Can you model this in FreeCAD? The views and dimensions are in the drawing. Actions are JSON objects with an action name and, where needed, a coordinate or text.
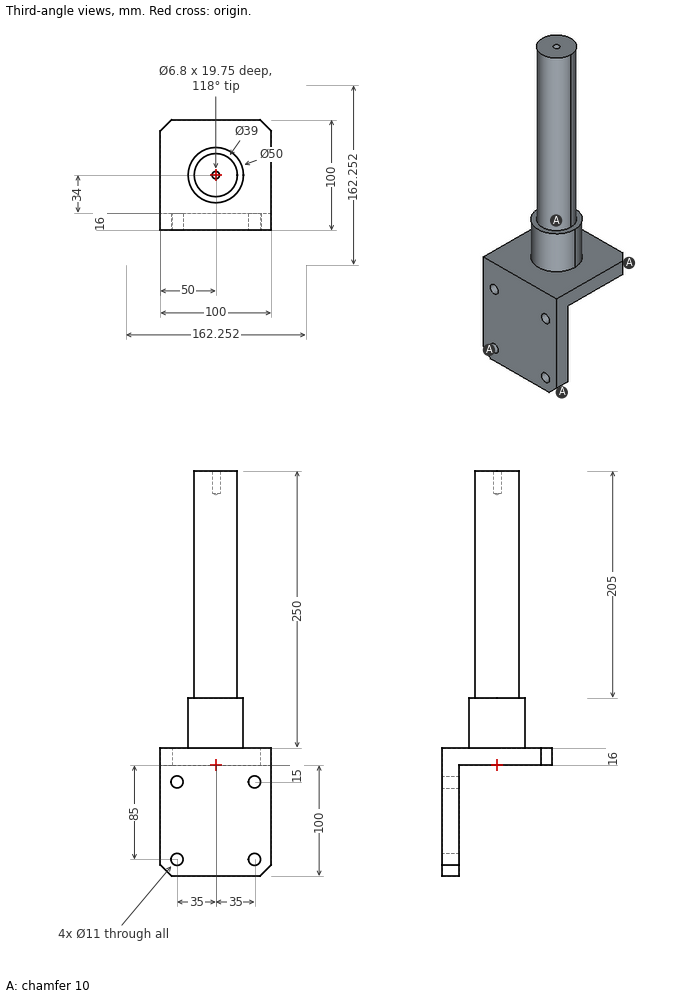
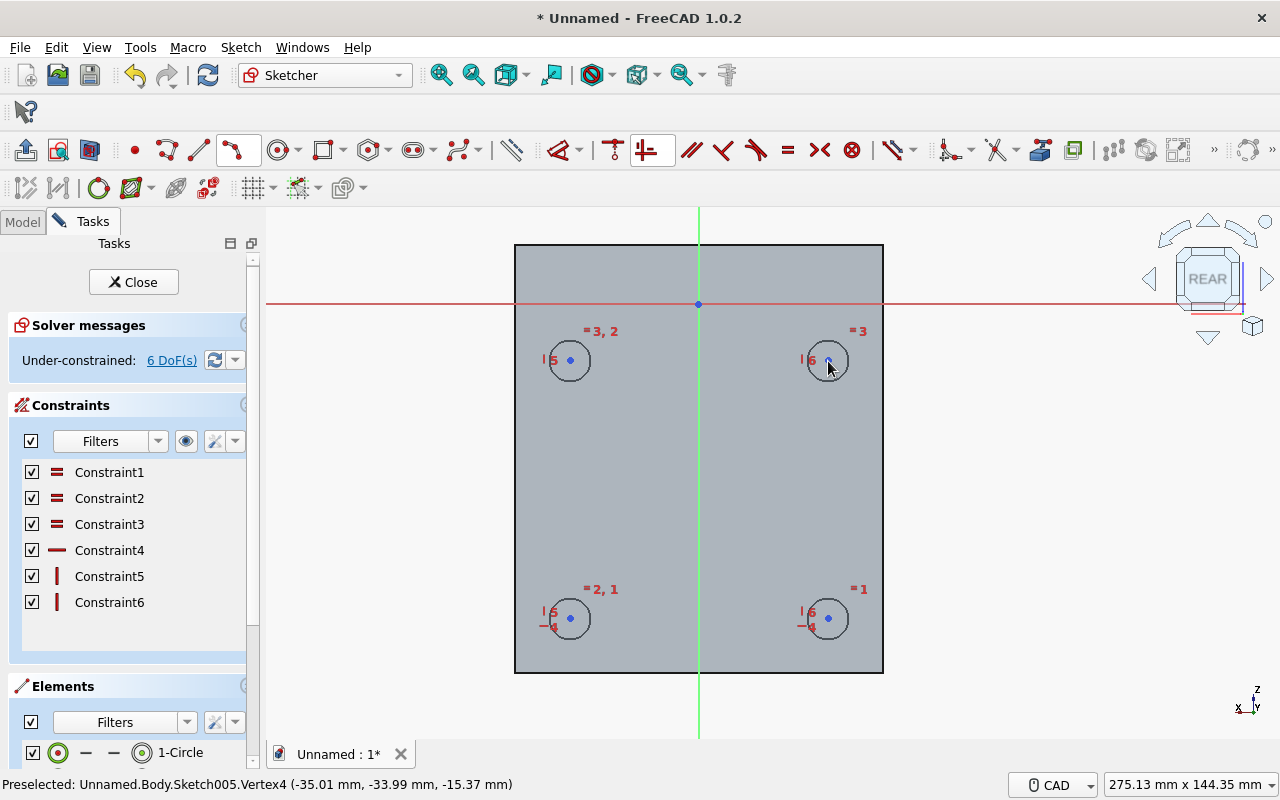
{"action": "left_click", "coordinate": [570, 361]}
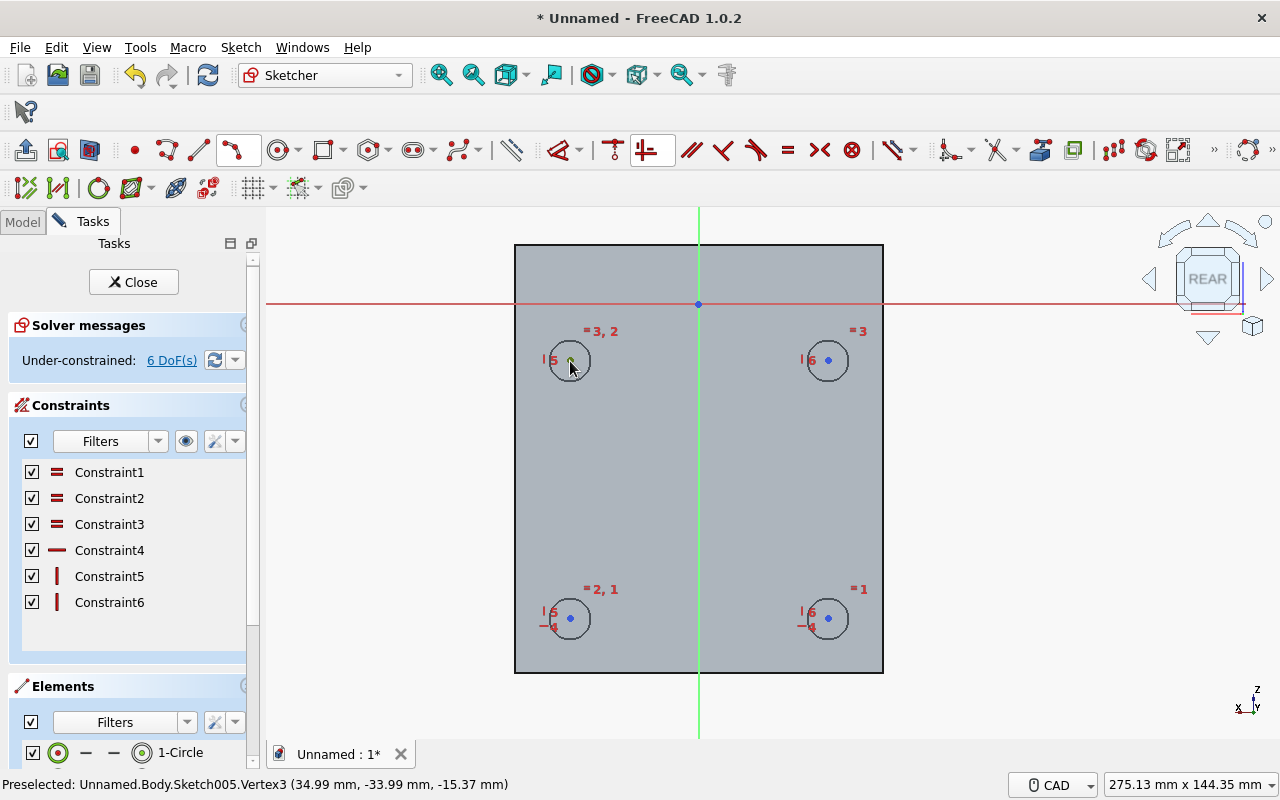
{"action": "left_click", "coordinate": [828, 361]}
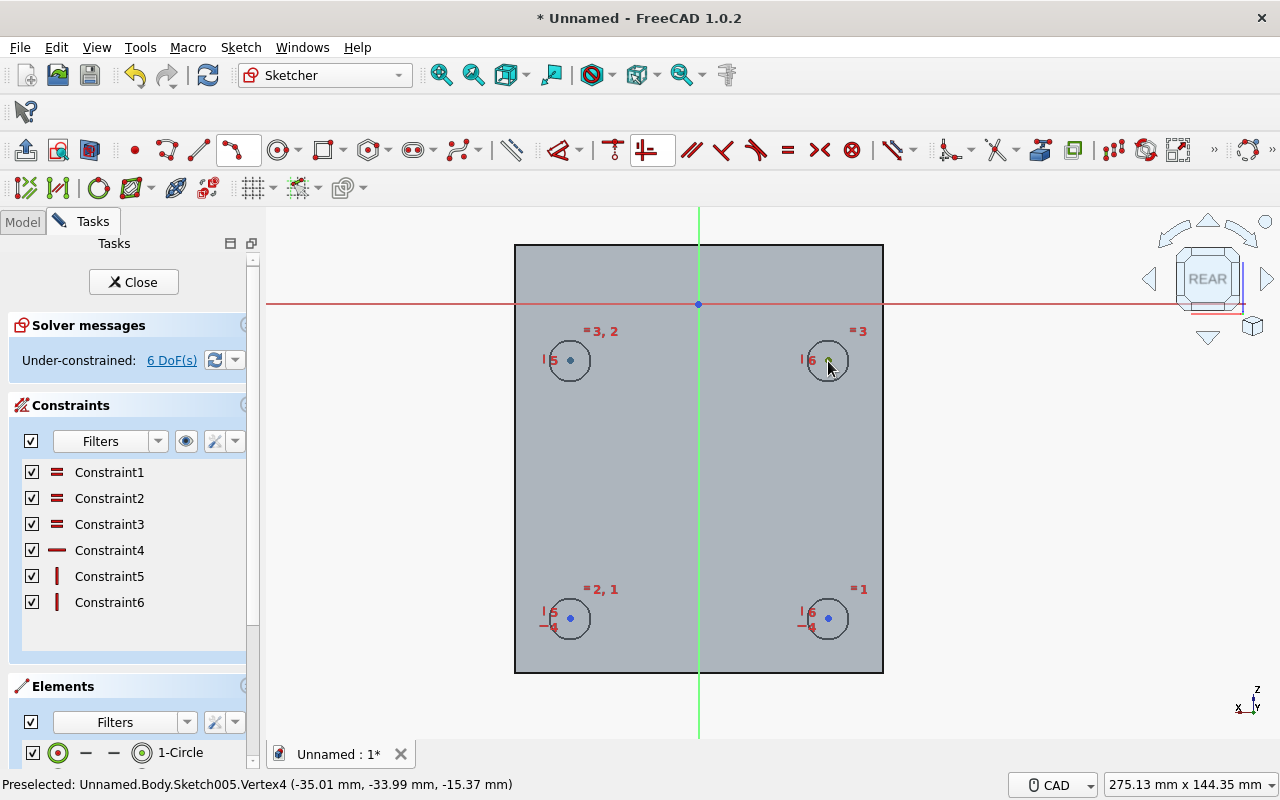
{"action": "key", "text": "h"}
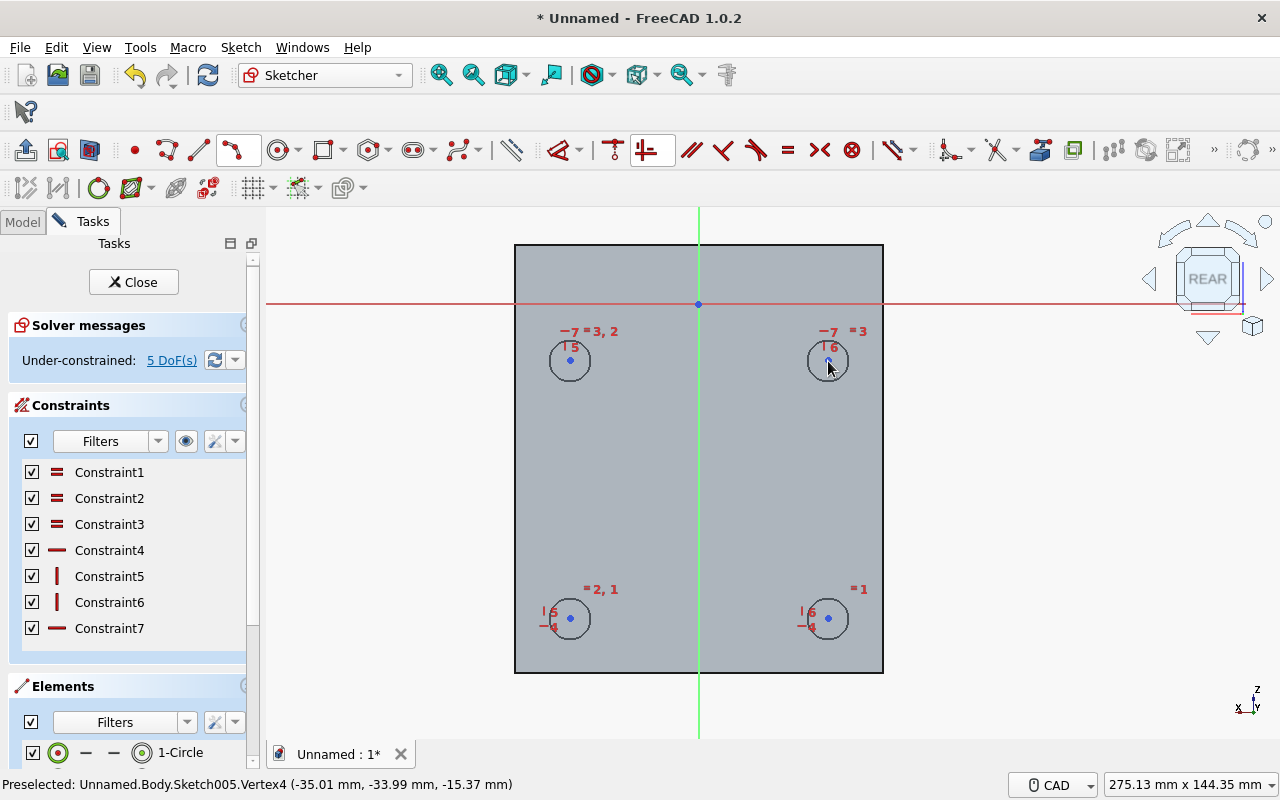
{"action": "left_click", "coordinate": [558, 150]}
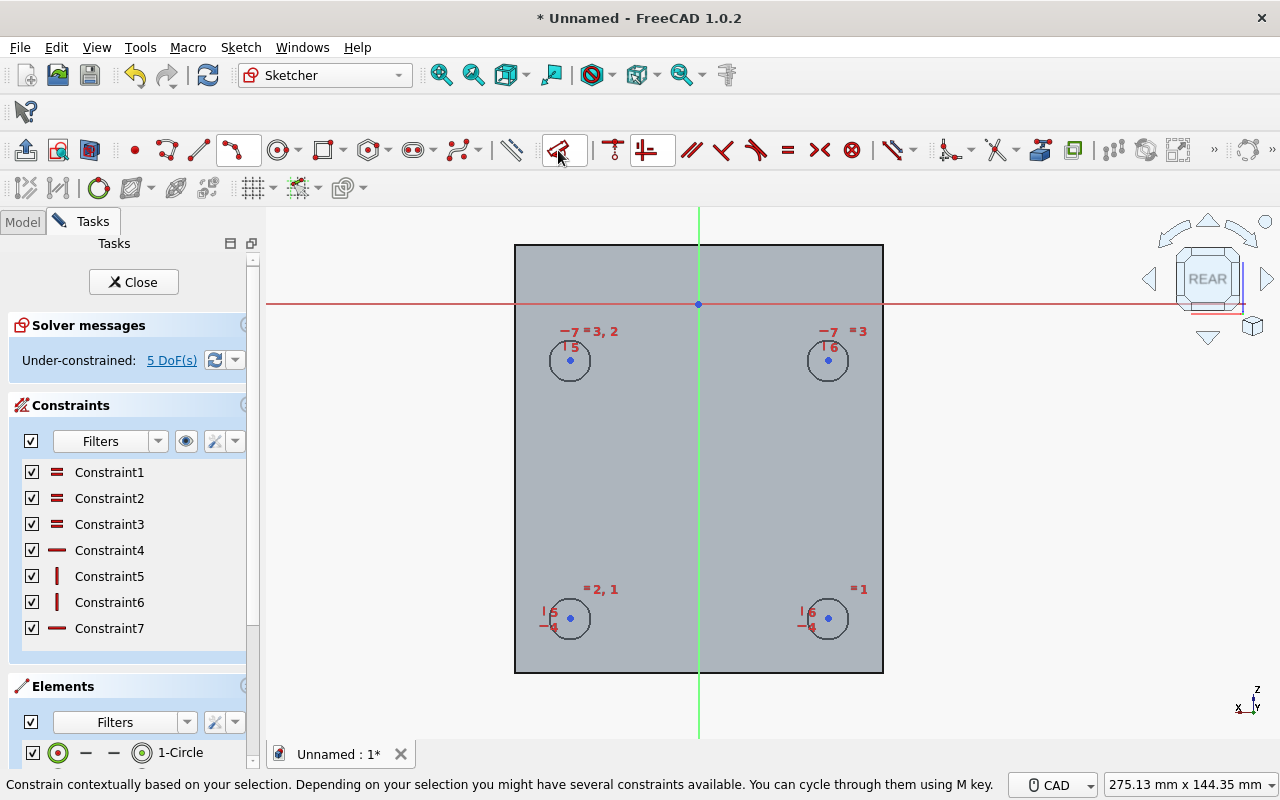
{"action": "left_click", "coordinate": [842, 604]}
{"action": "left_click", "coordinate": [864, 581]}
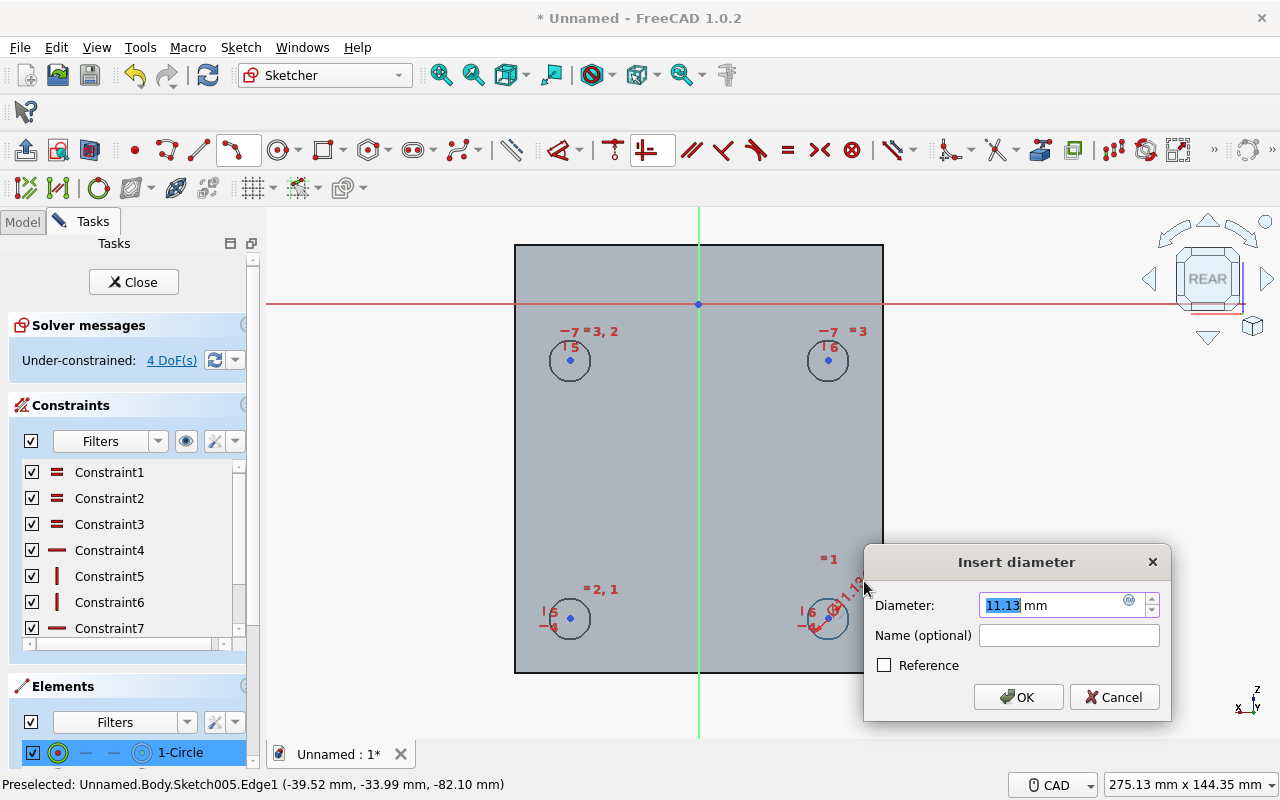
{"action": "type", "text": "11"}
{"action": "key", "text": "Return"}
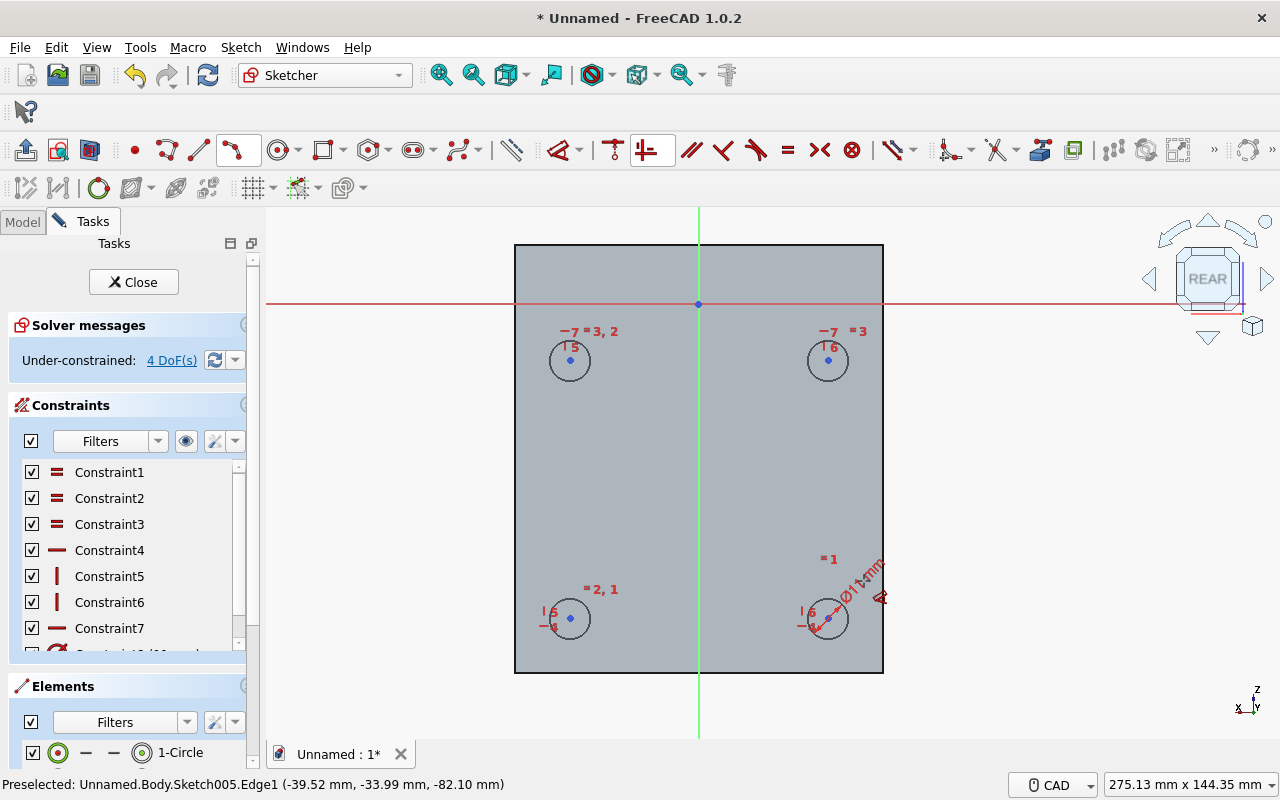
{"action": "left_click", "coordinate": [828, 619]}
{"action": "left_click", "coordinate": [763, 270]}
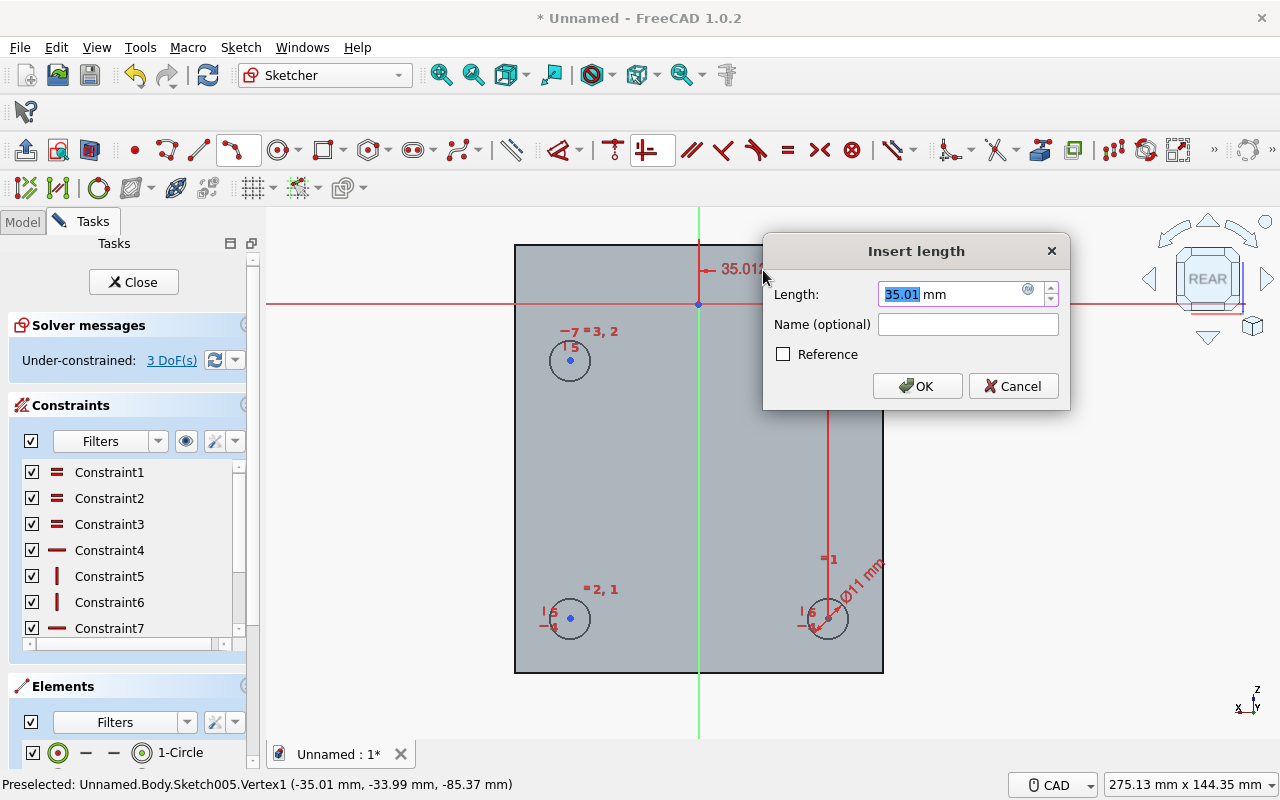
{"action": "type", "text": "35"}
{"action": "key", "text": "Return"}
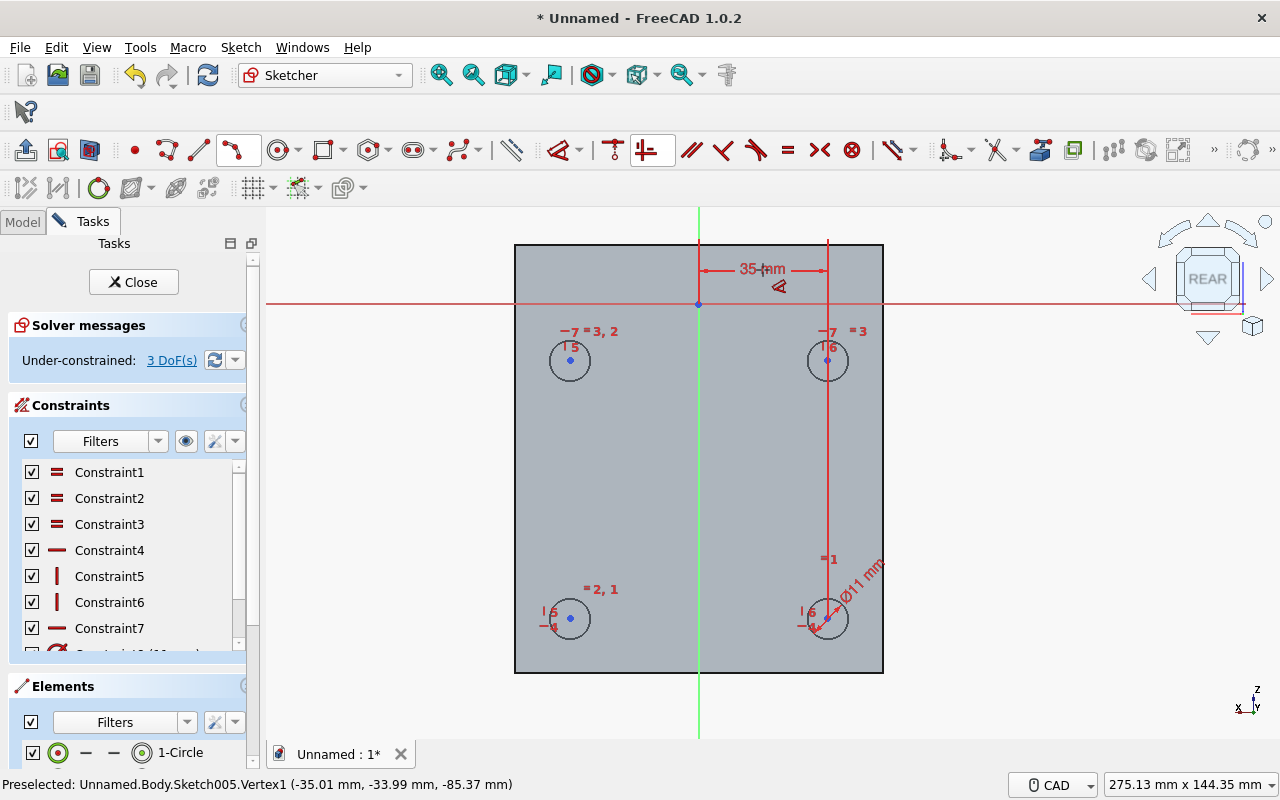
{"action": "left_click", "coordinate": [828, 619]}
{"action": "left_click", "coordinate": [862, 462]}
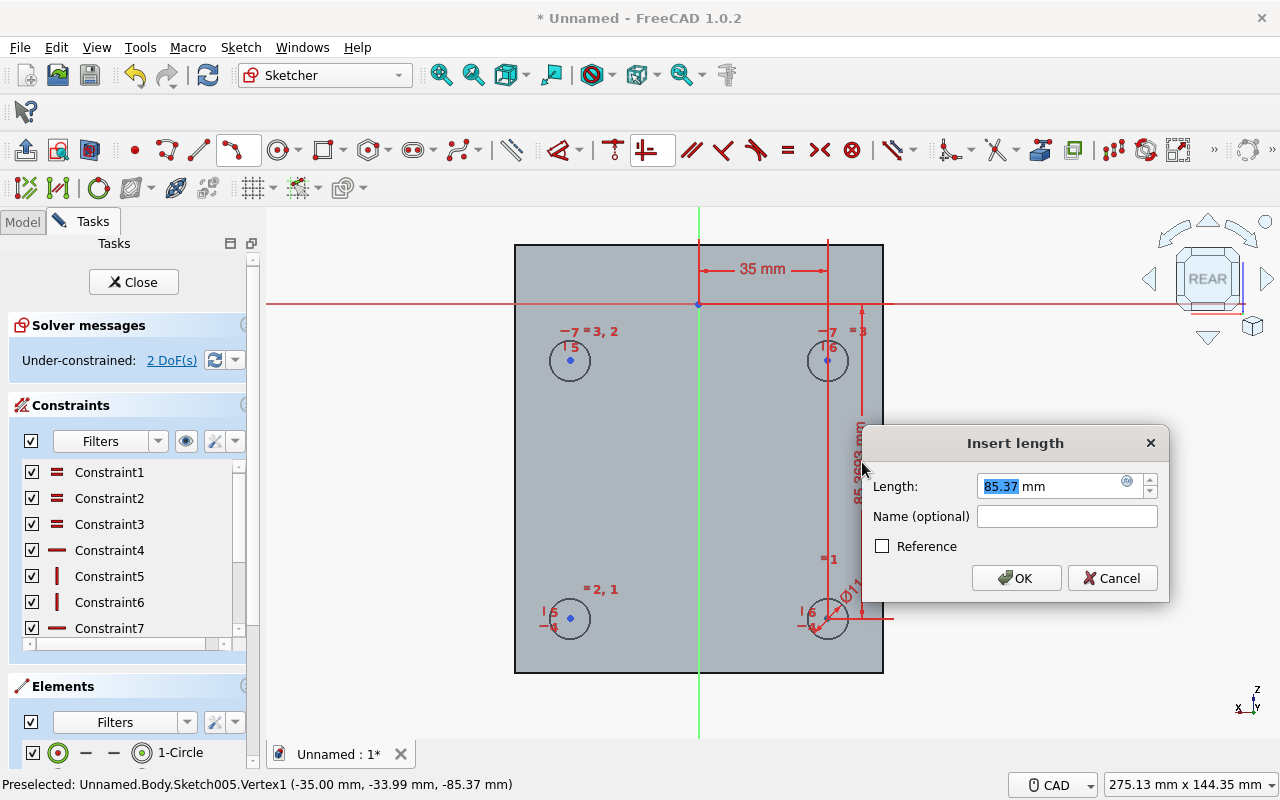
{"action": "type", "text": "85"}
{"action": "key", "text": "Return"}